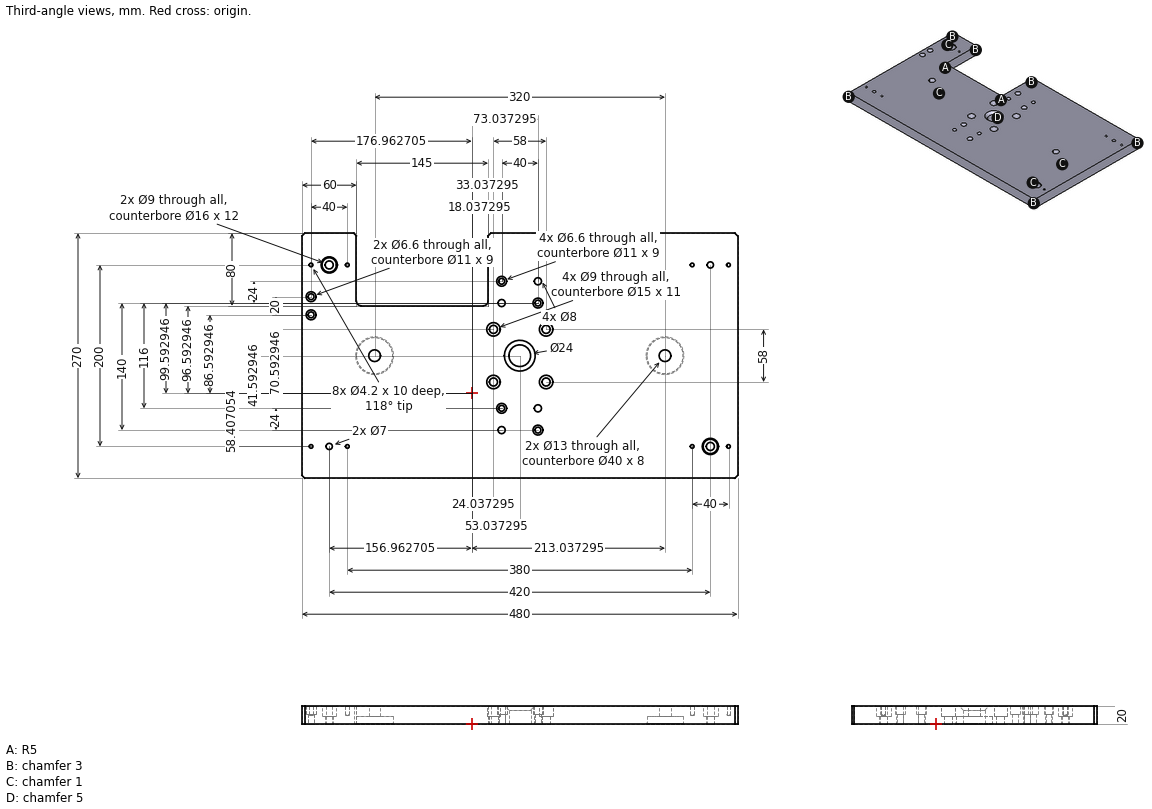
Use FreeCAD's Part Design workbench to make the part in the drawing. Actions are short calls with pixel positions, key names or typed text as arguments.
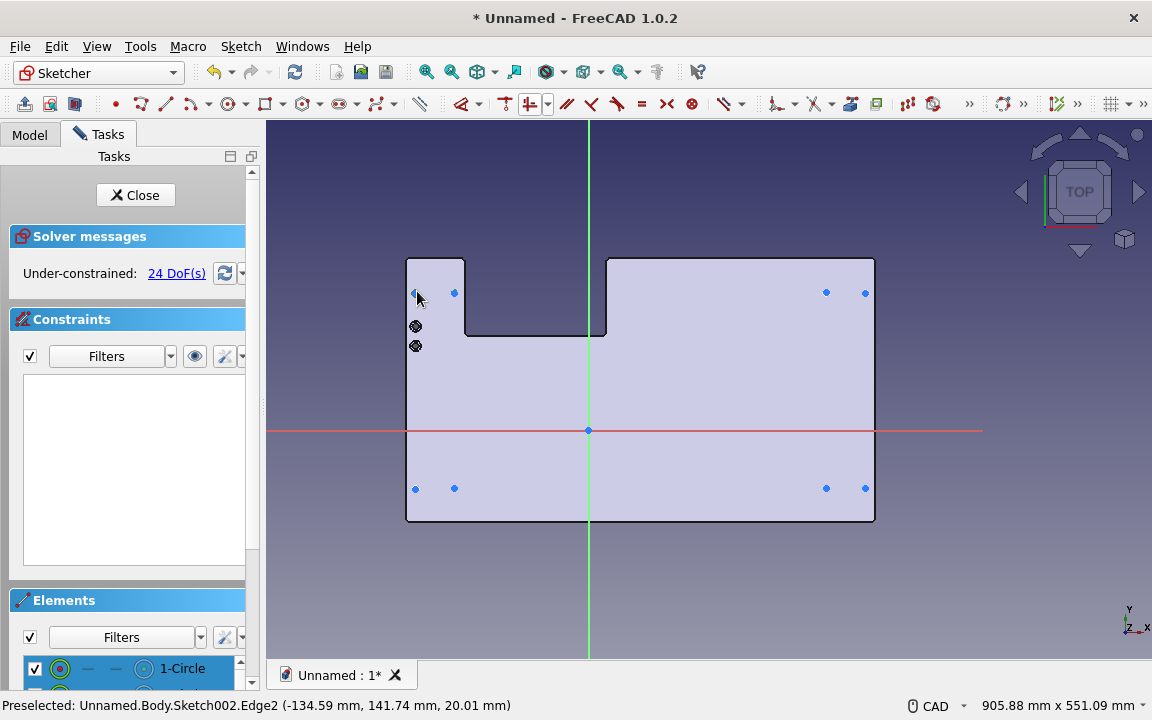
scroll(418, 487, up, 8)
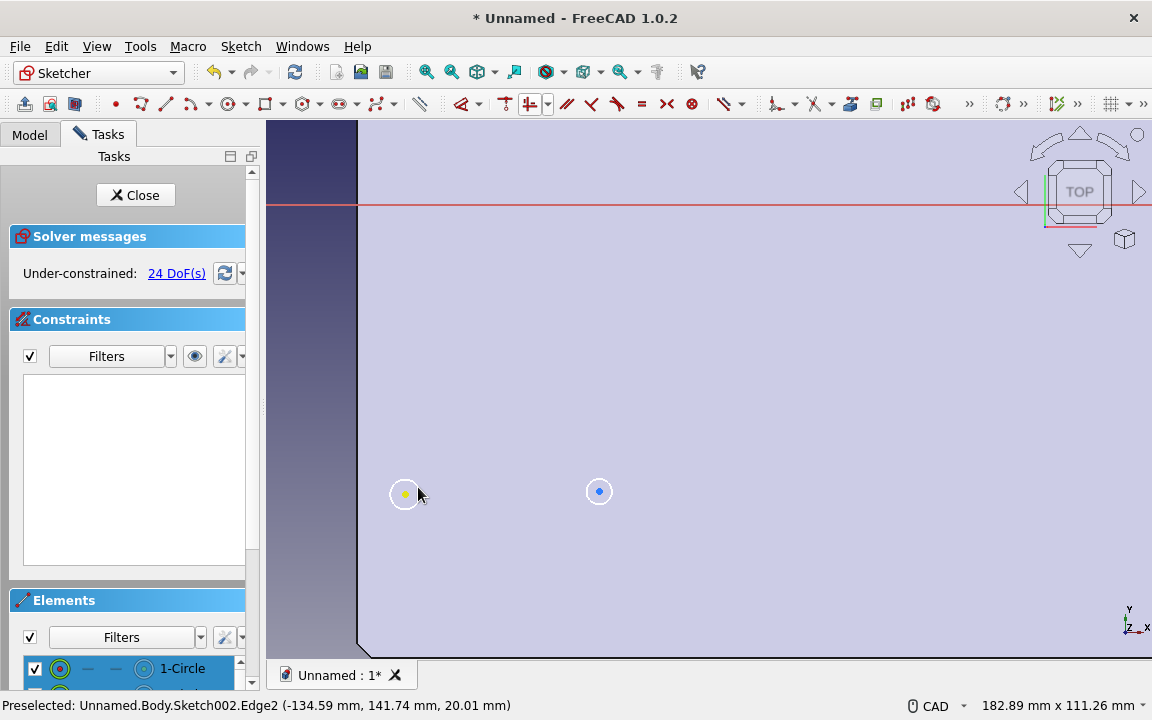
click(416, 484)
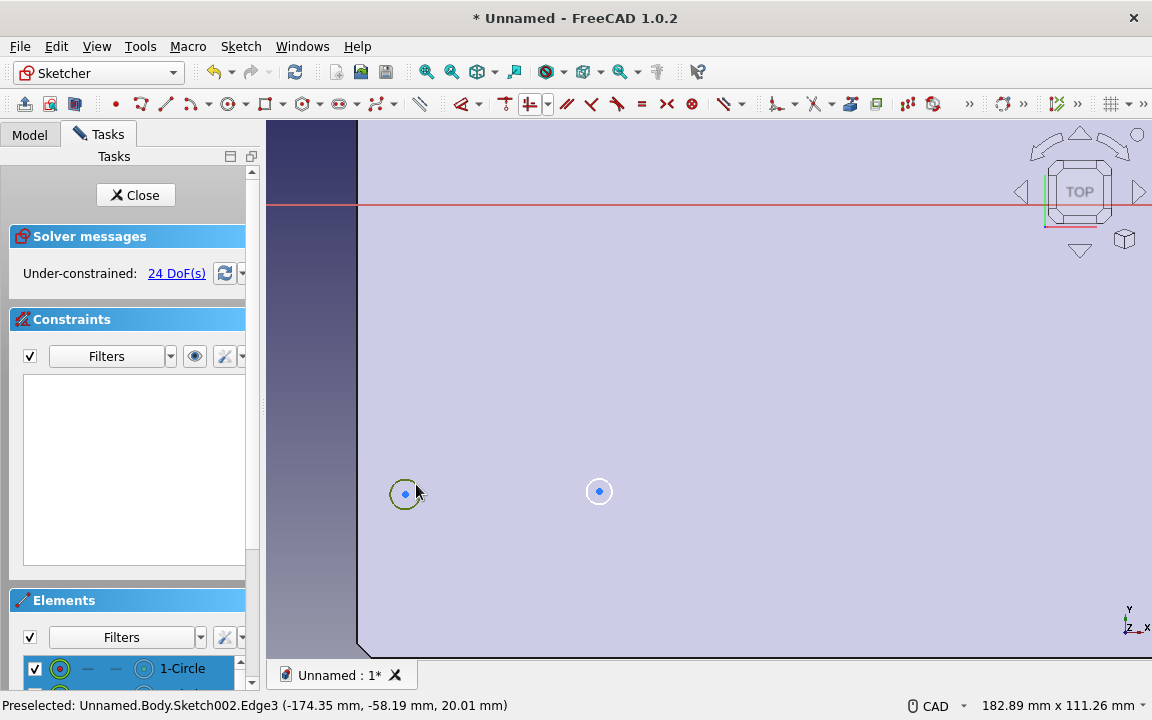
click(608, 483)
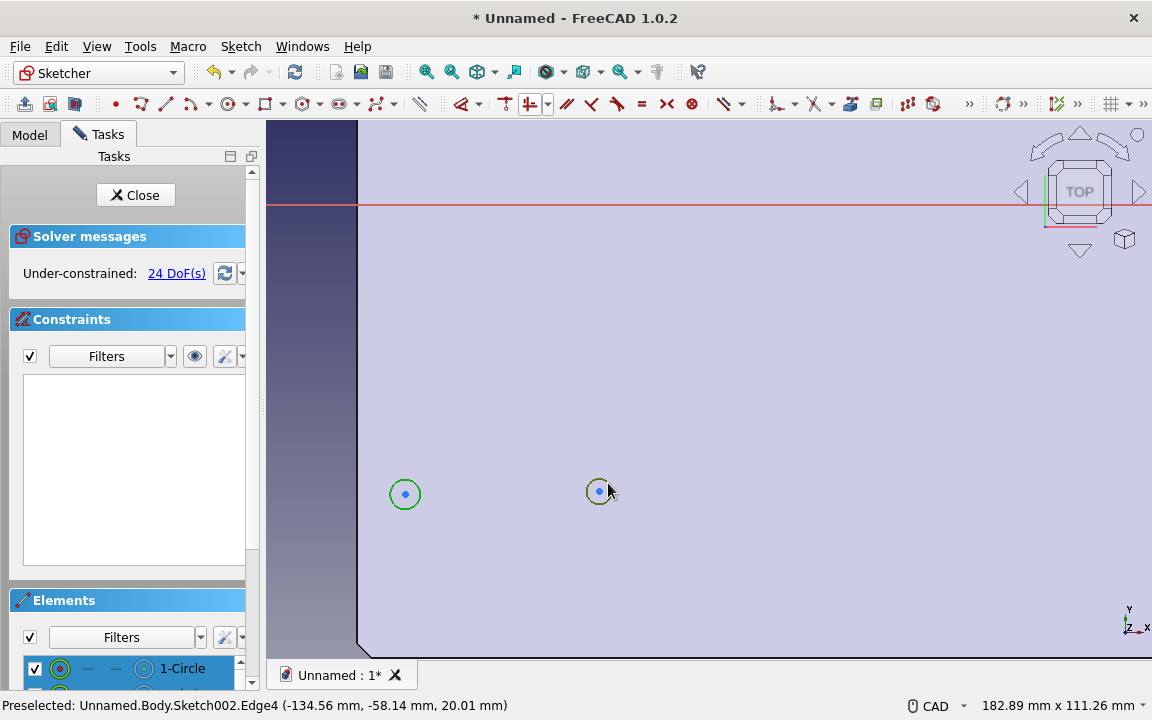
scroll(418, 487, down, 8)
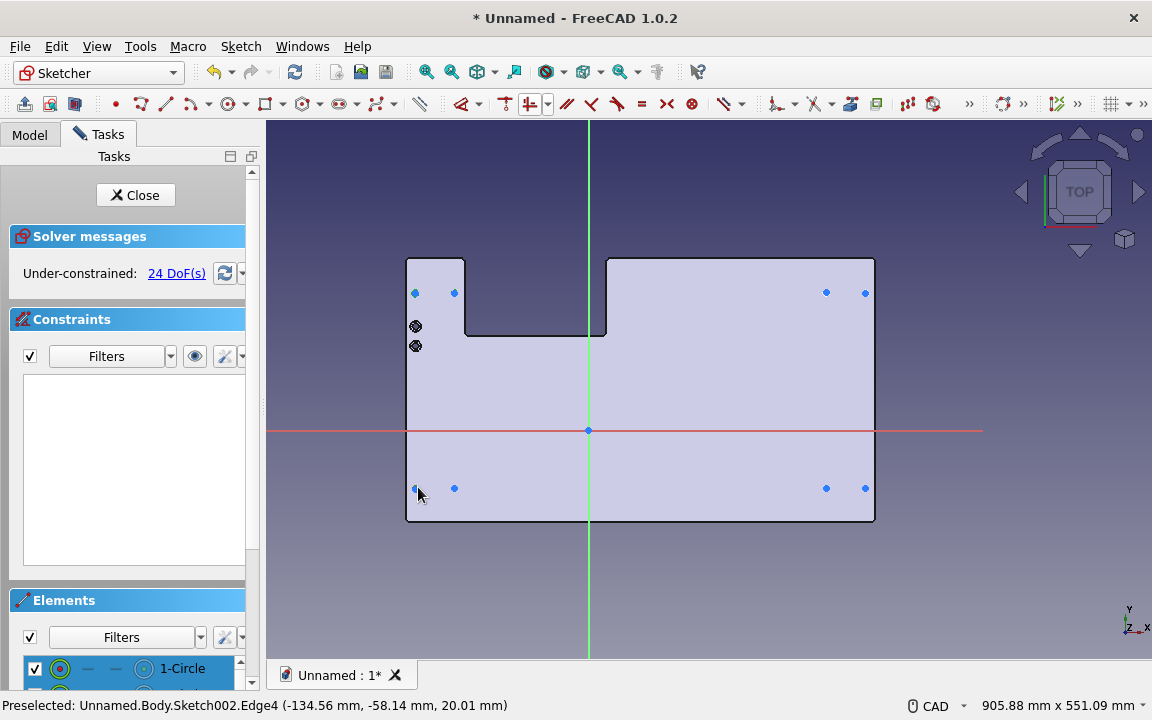
scroll(828, 487, up, 9)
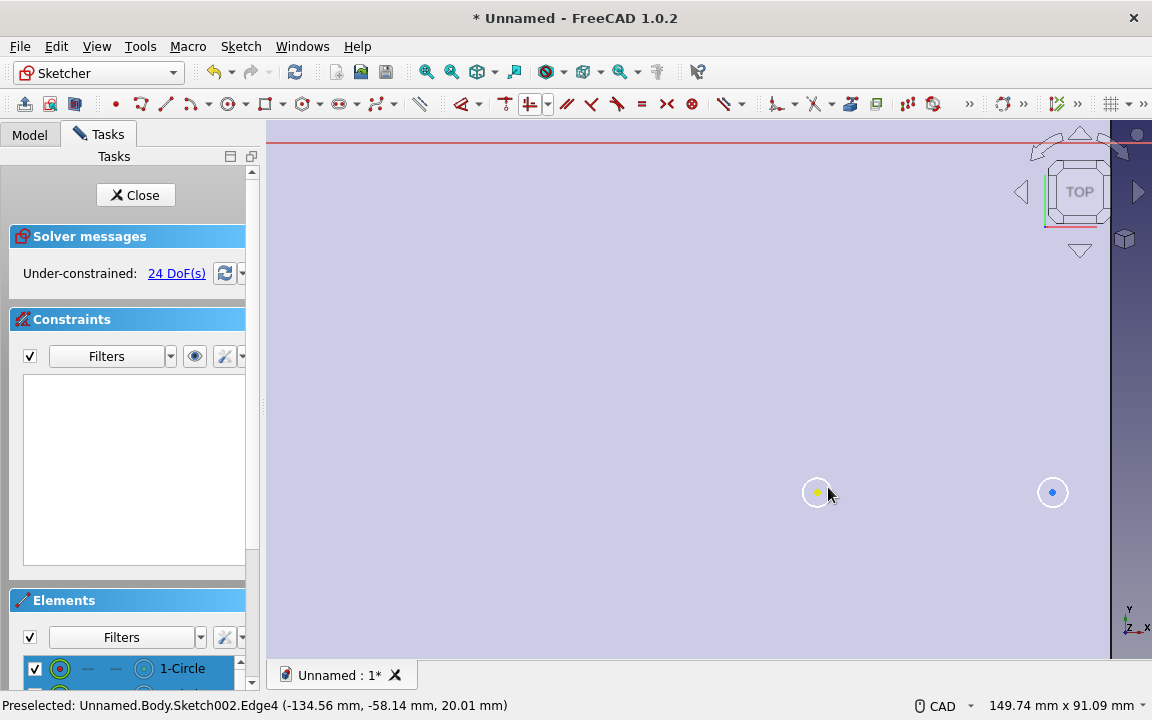
click(827, 482)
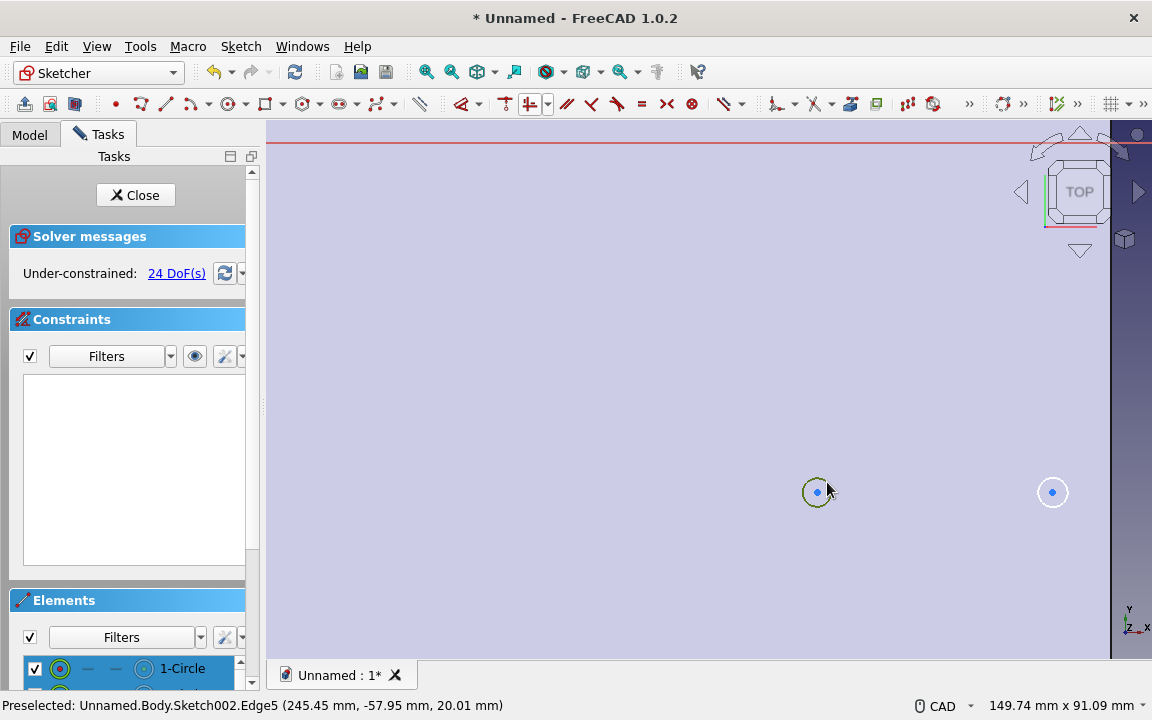
scroll(829, 487, down, 9)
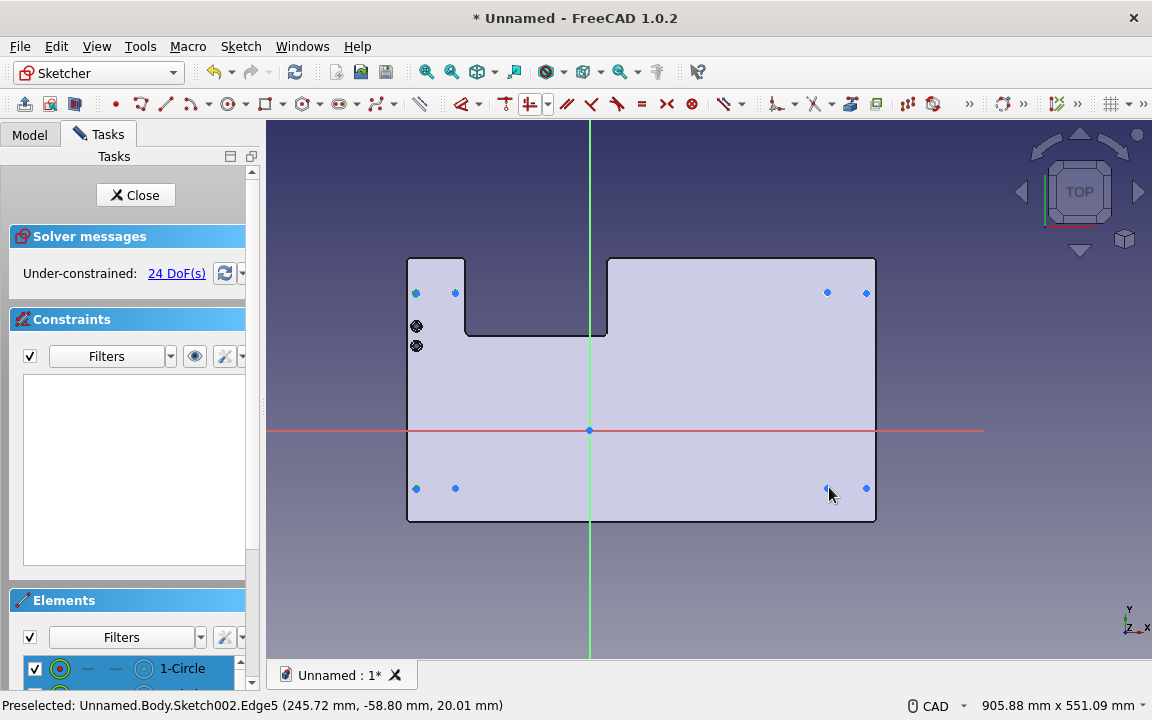
scroll(868, 487, up, 9)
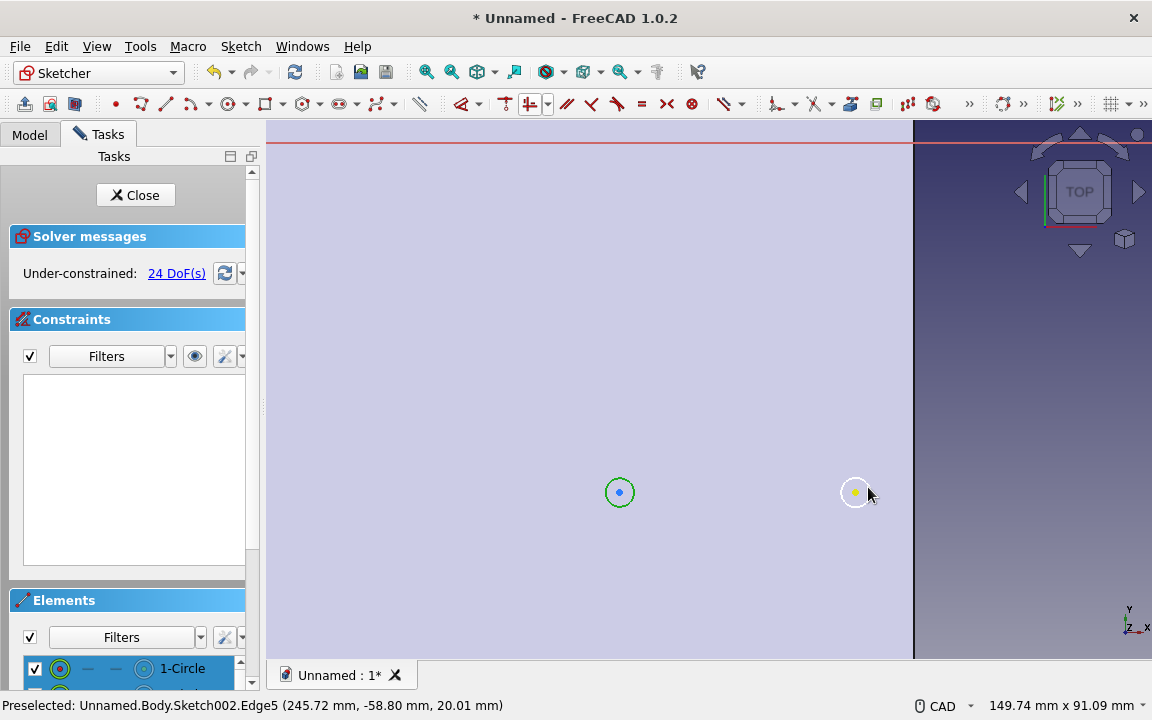
click(866, 482)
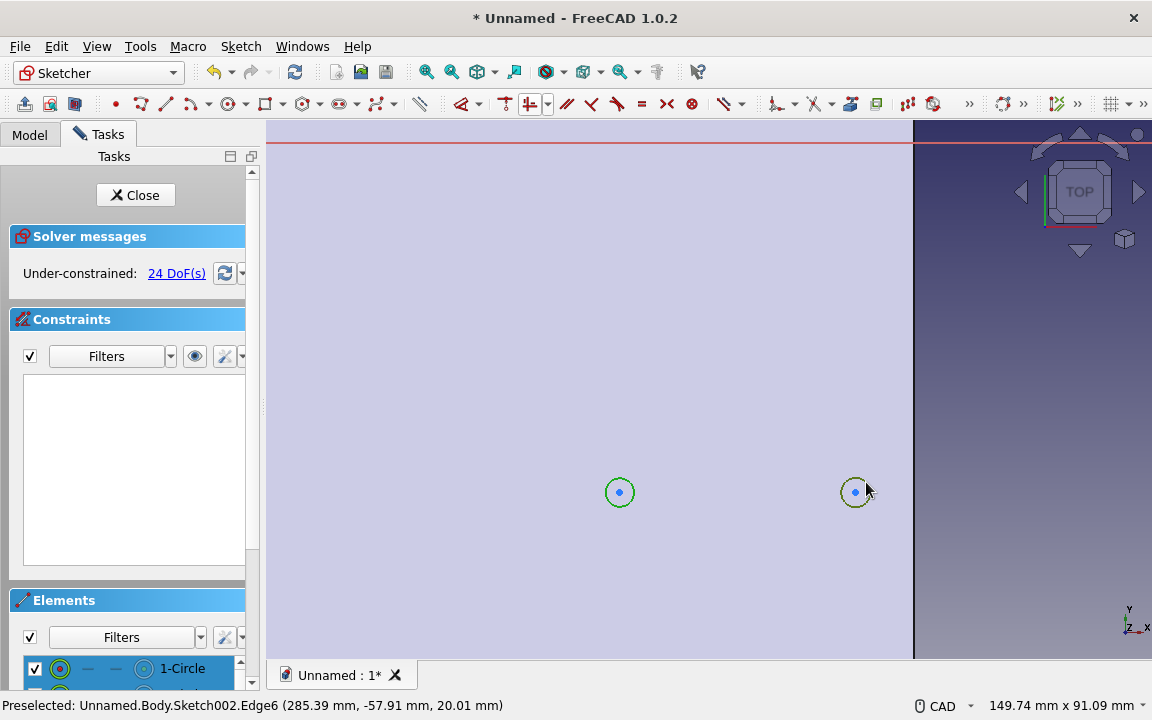
scroll(868, 487, down, 9)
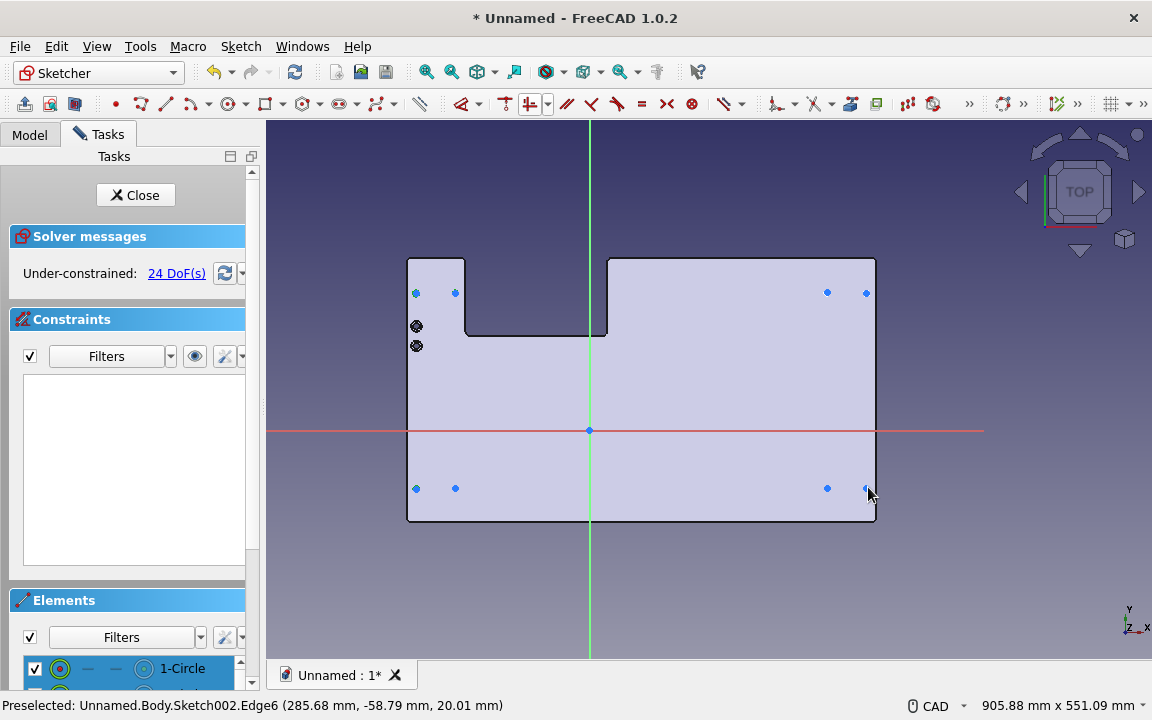
scroll(869, 291, up, 8)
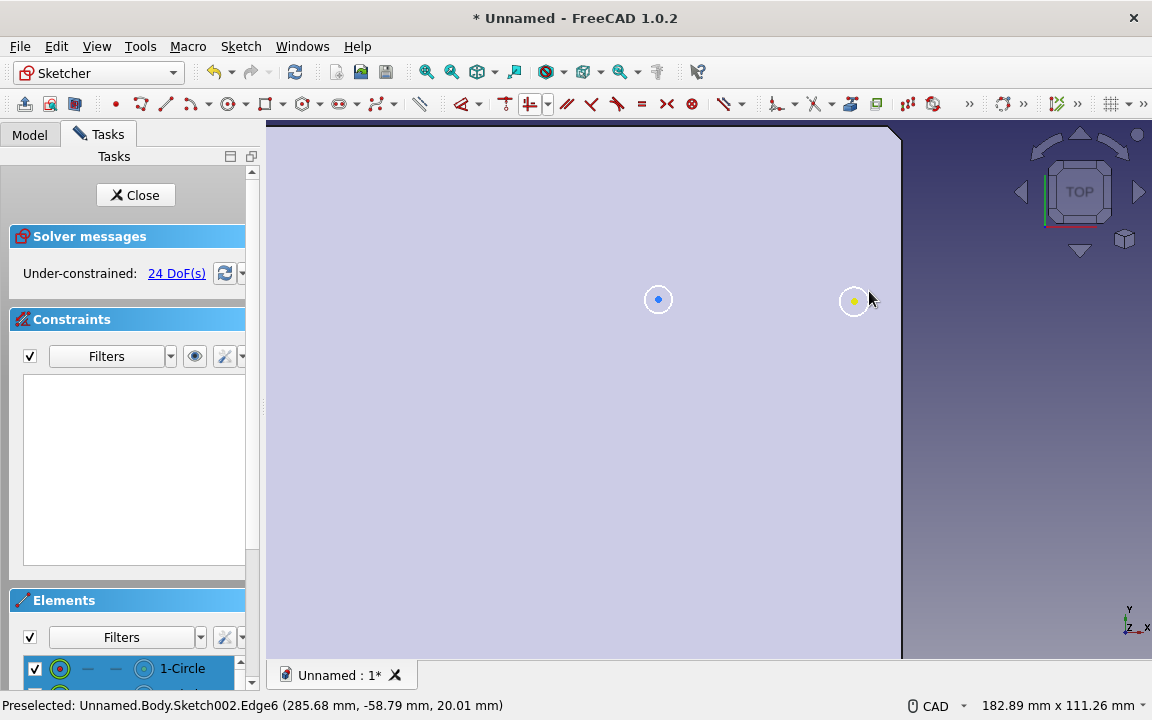
click(864, 292)